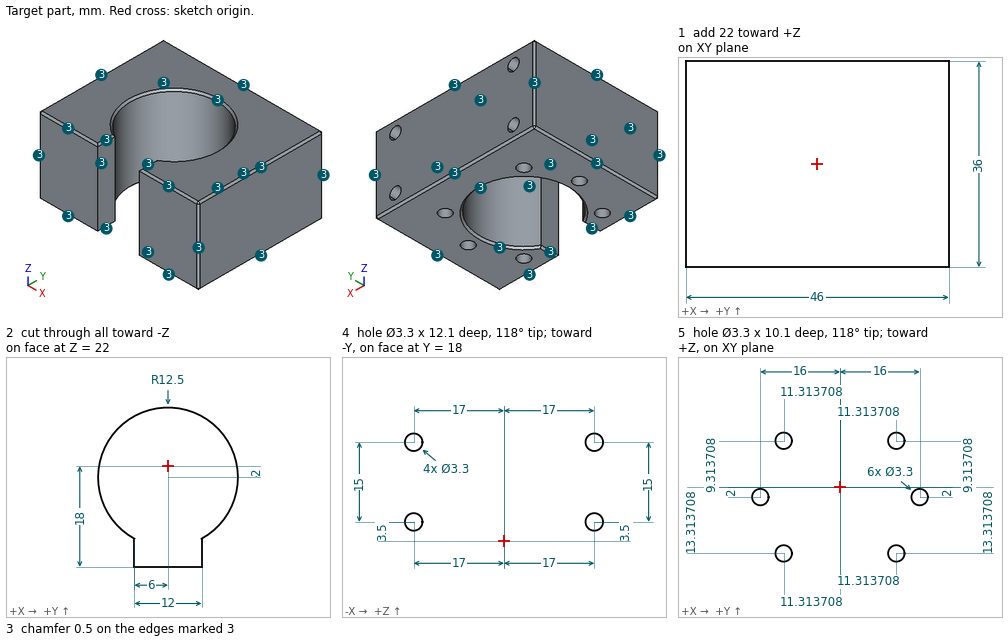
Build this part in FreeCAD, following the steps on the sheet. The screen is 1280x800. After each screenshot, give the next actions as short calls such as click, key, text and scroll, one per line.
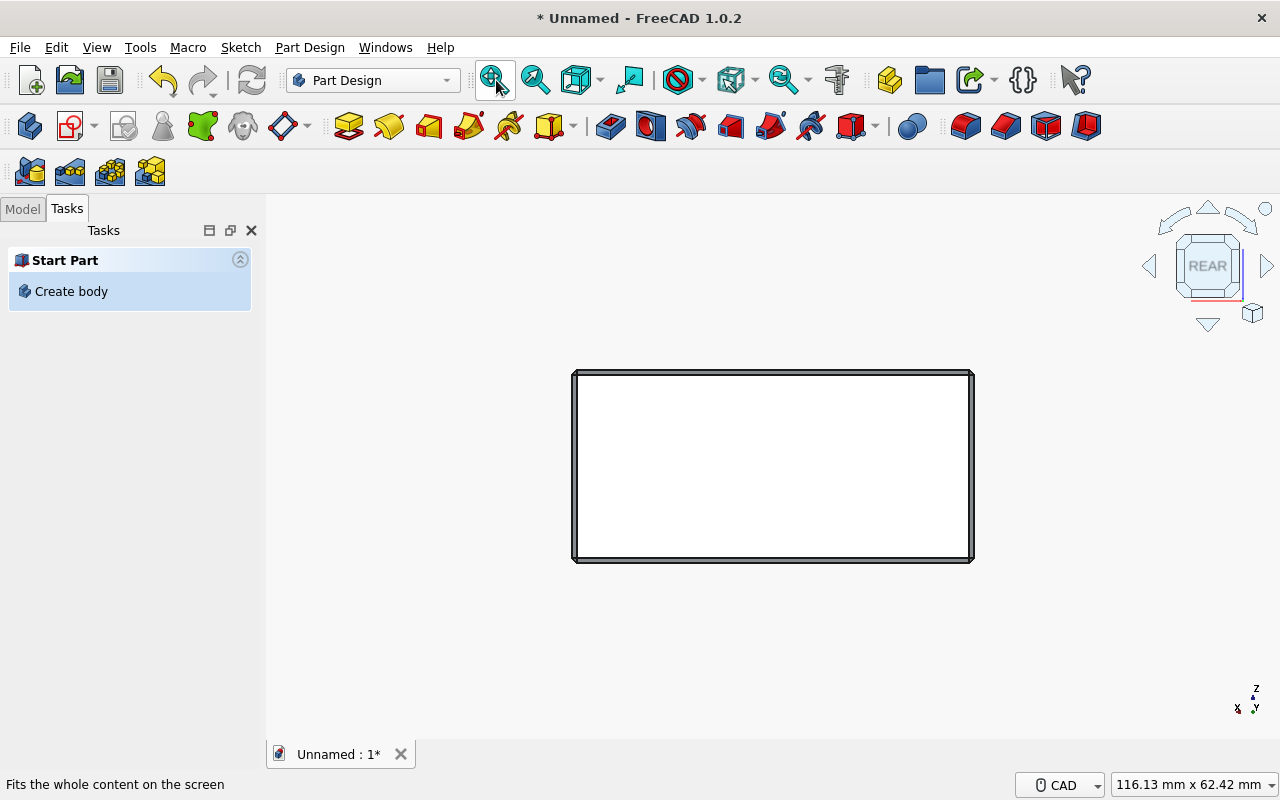
click(717, 466)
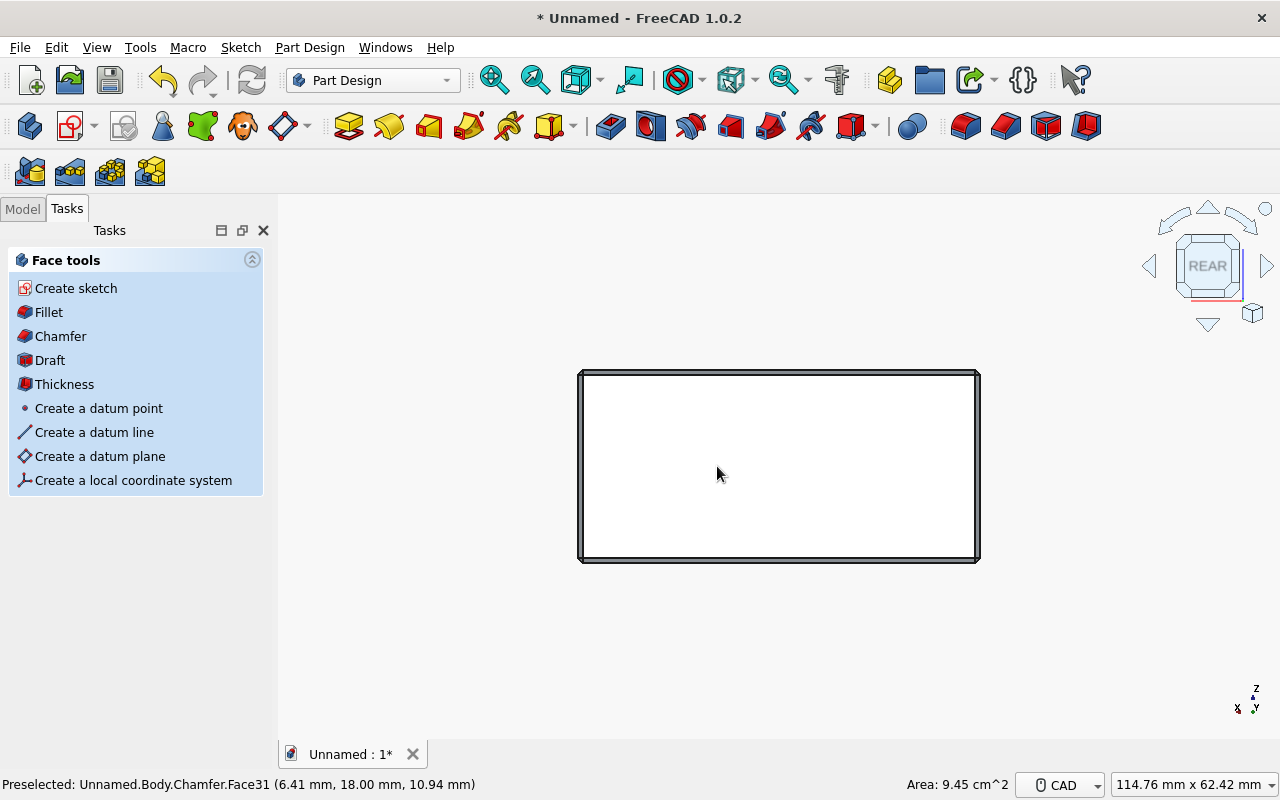
click(70, 126)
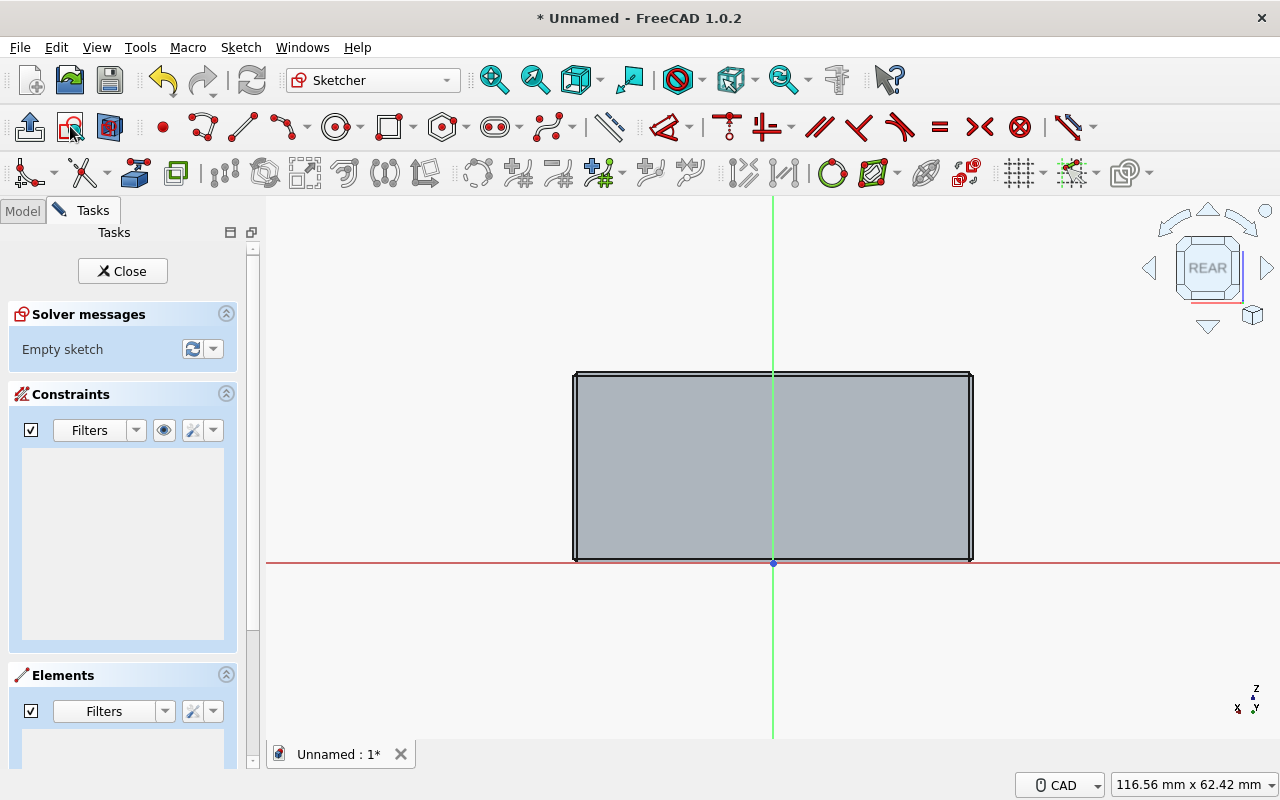
scroll(856, 485, up, 3)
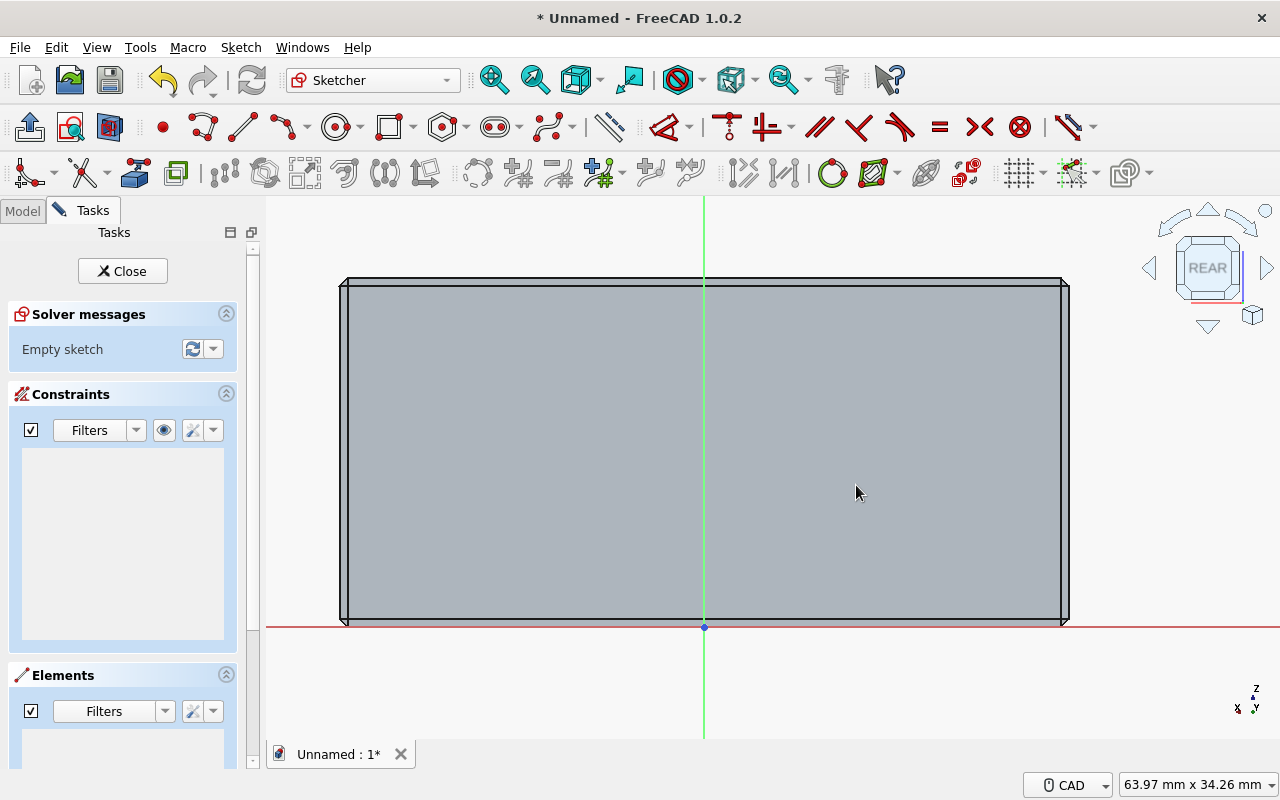
click(336, 128)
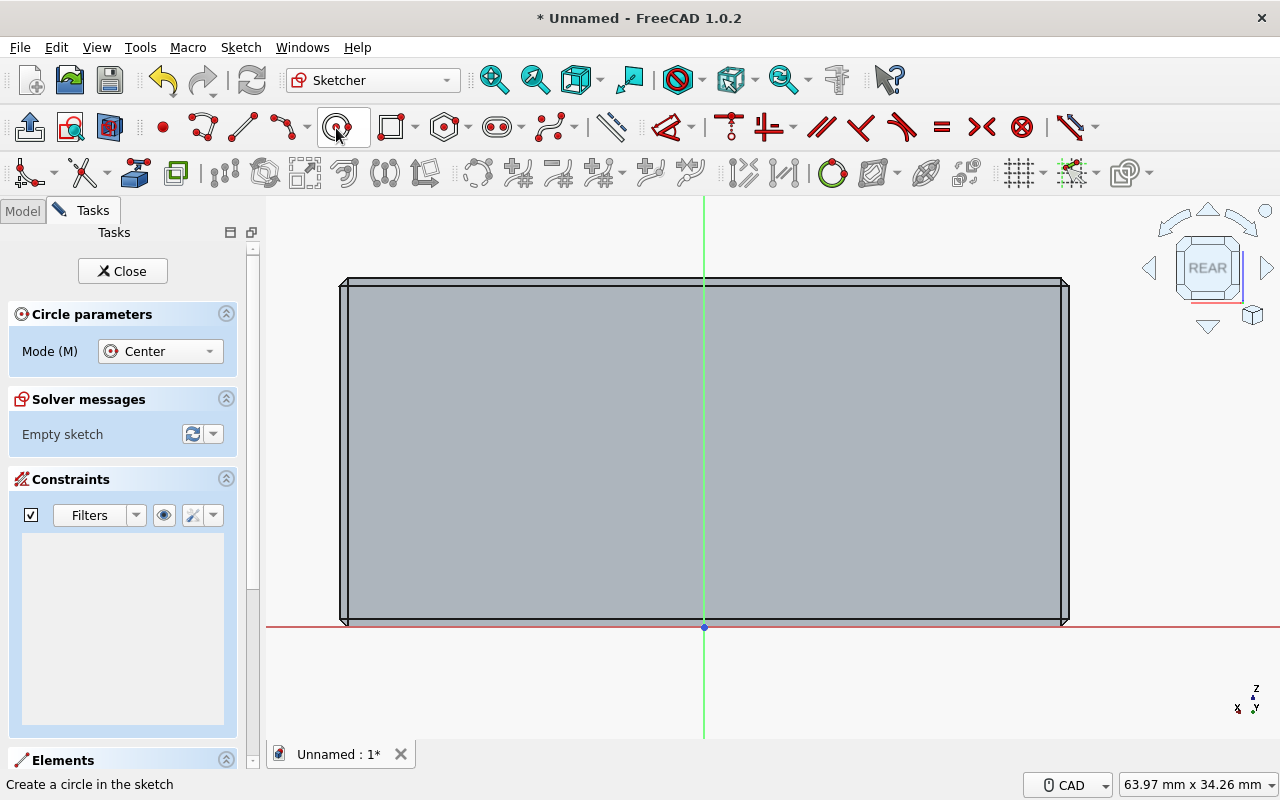
click(435, 334)
move(453, 315)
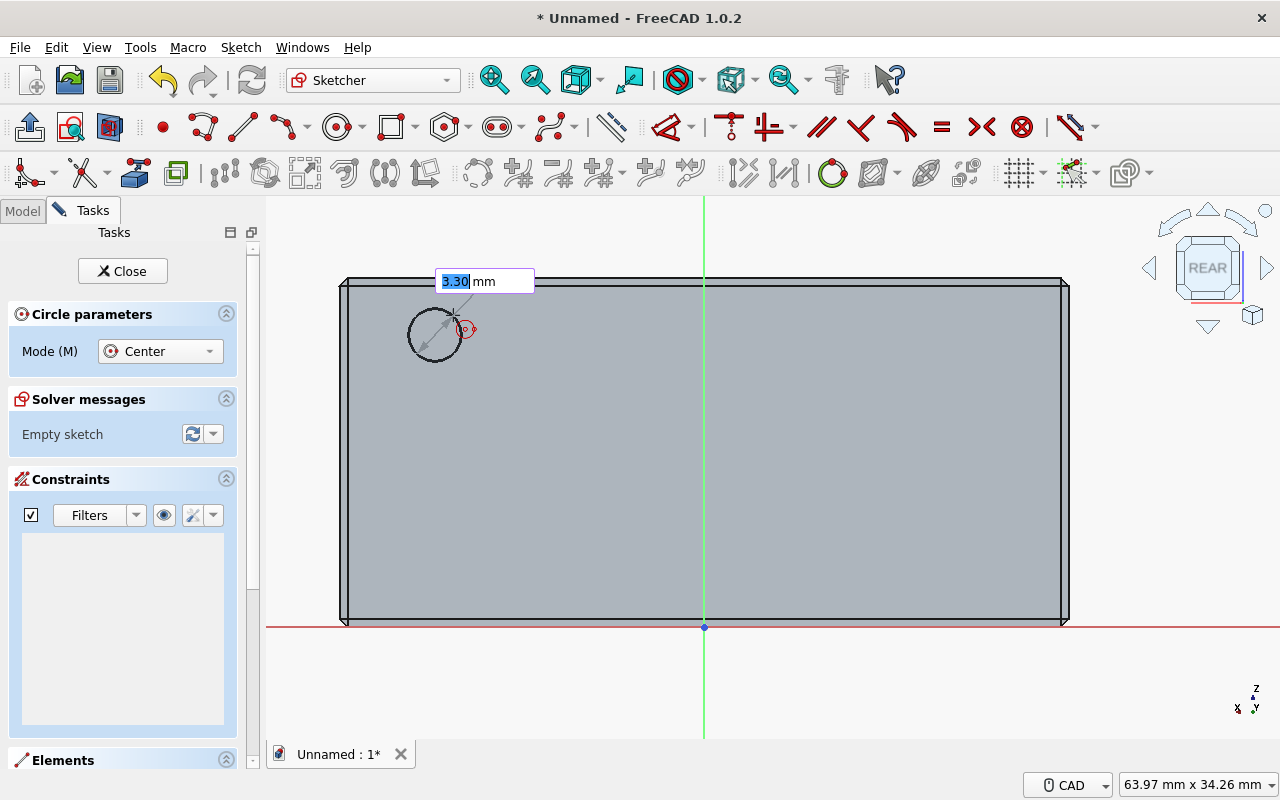
text(3.3)
key(Return)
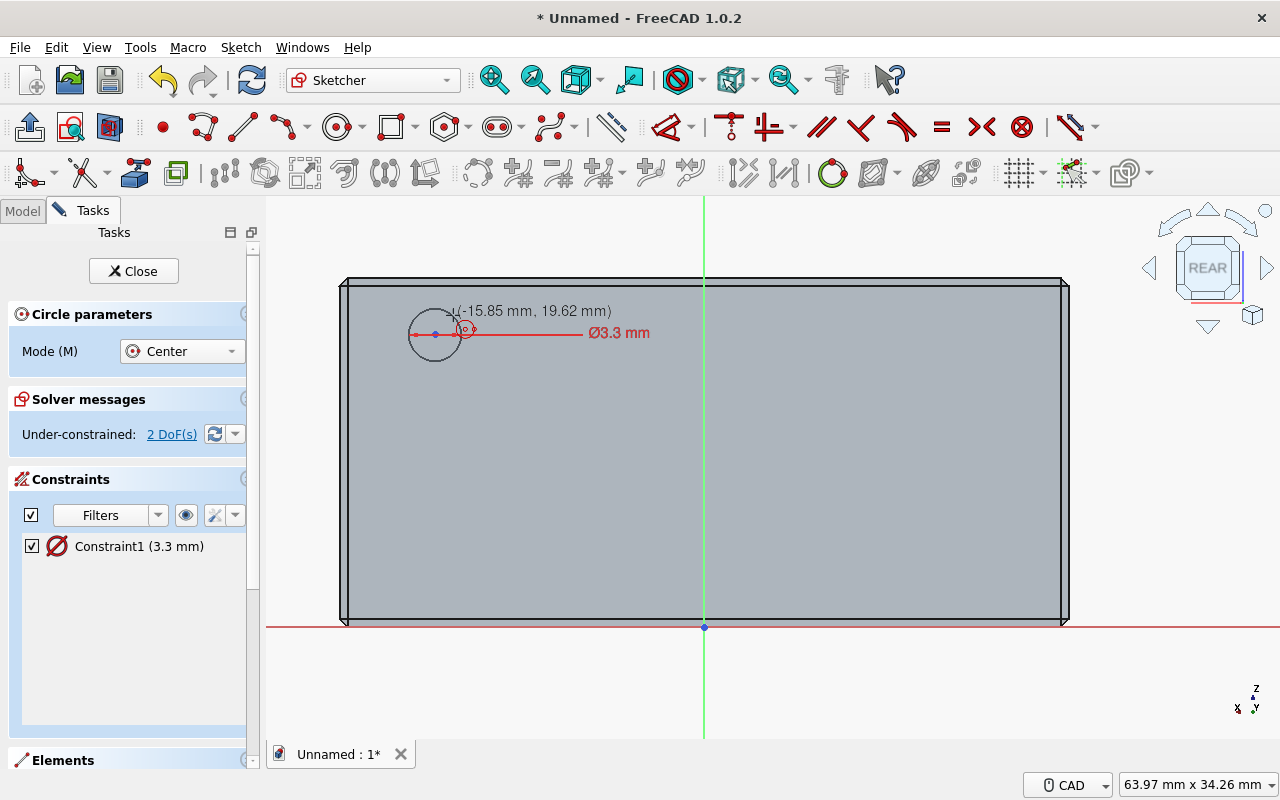
click(435, 572)
move(453, 553)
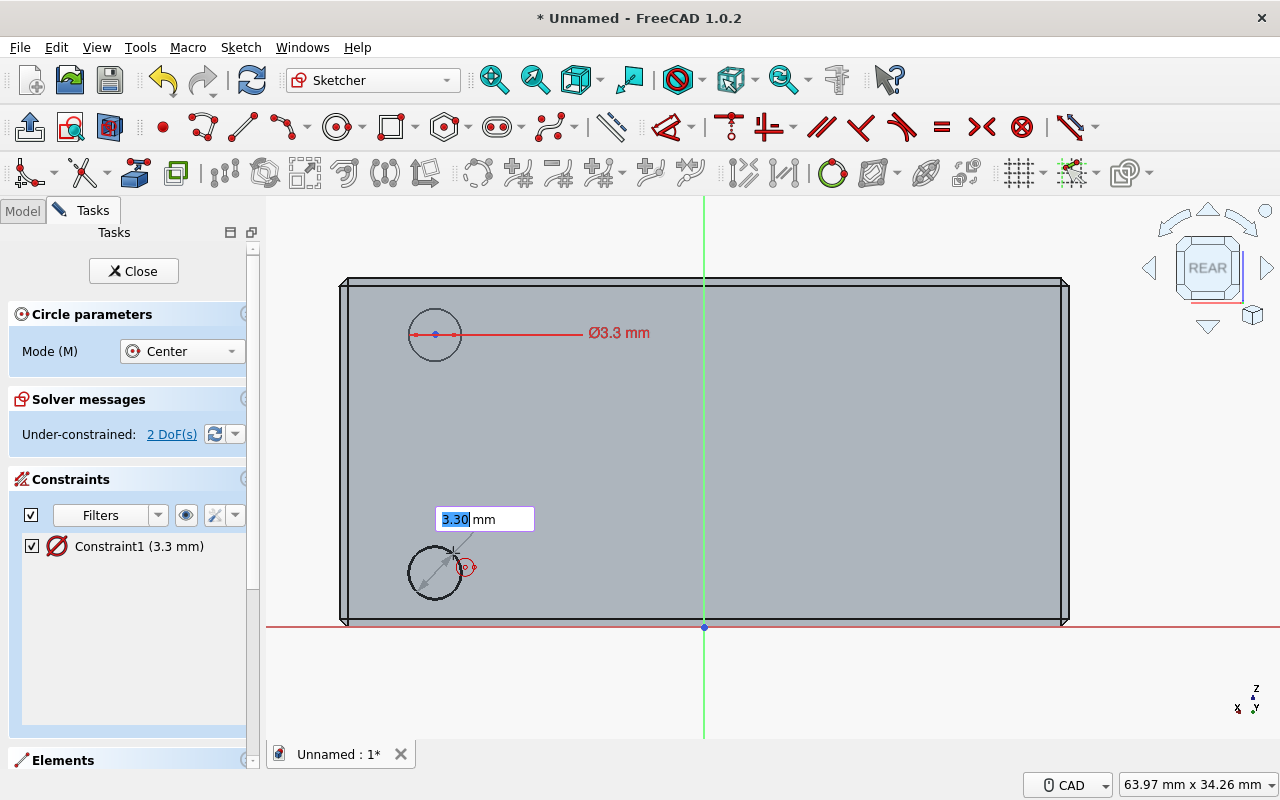
text(3.3)
key(Return)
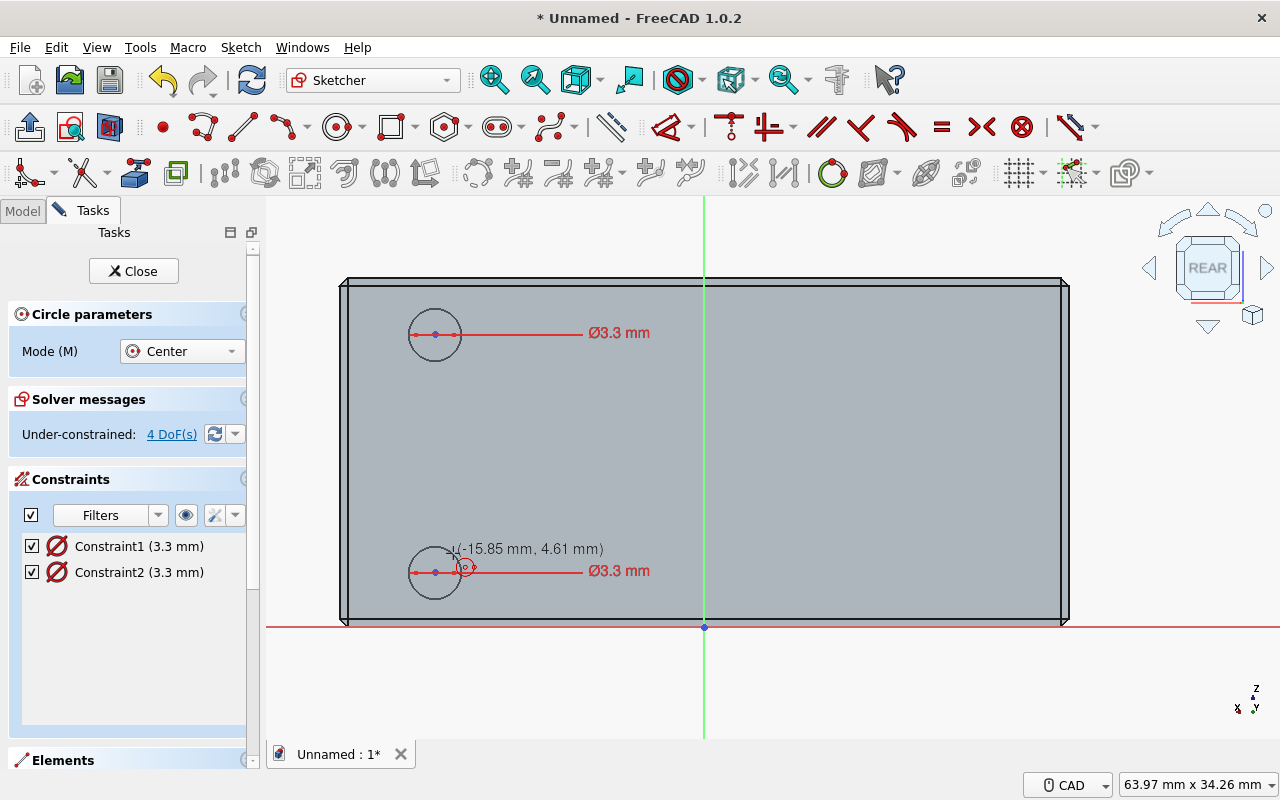
click(974, 572)
move(992, 553)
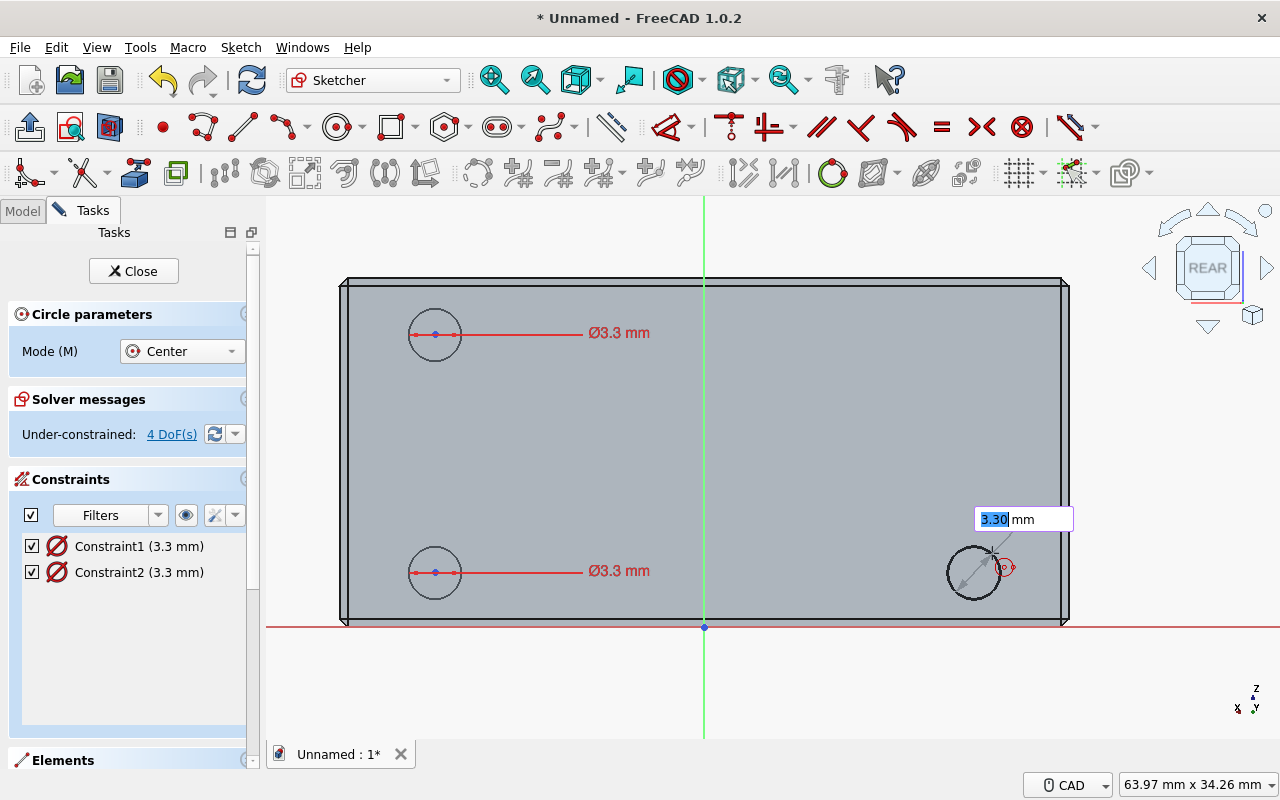
text(3.3)
key(Return)